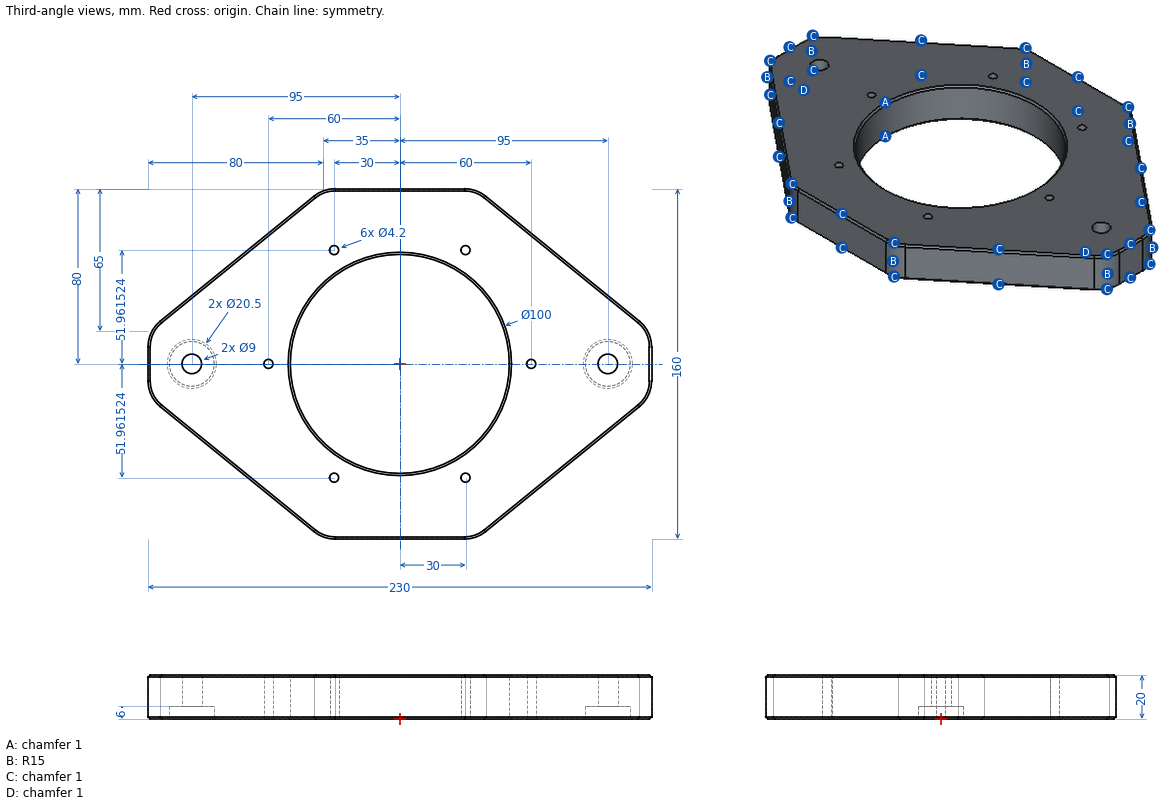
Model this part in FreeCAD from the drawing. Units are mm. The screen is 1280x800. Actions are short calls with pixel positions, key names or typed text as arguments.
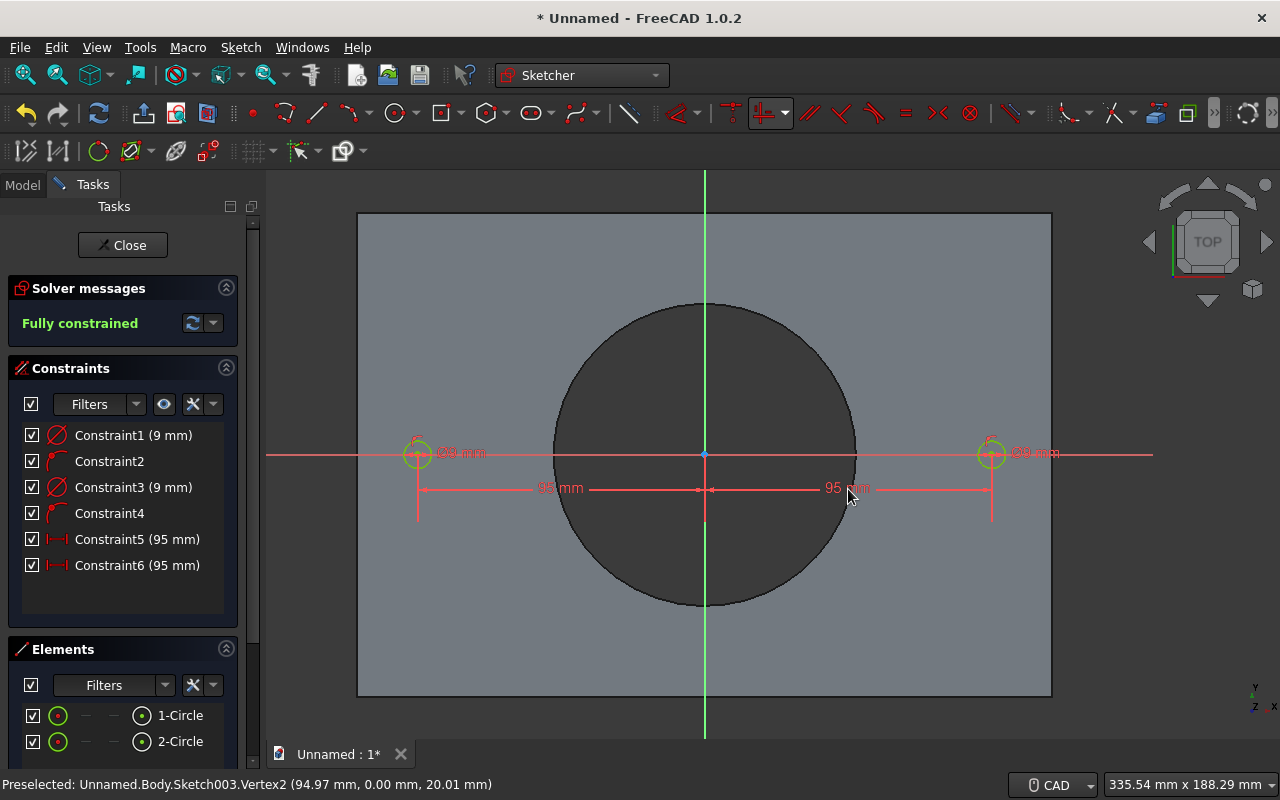
click(123, 245)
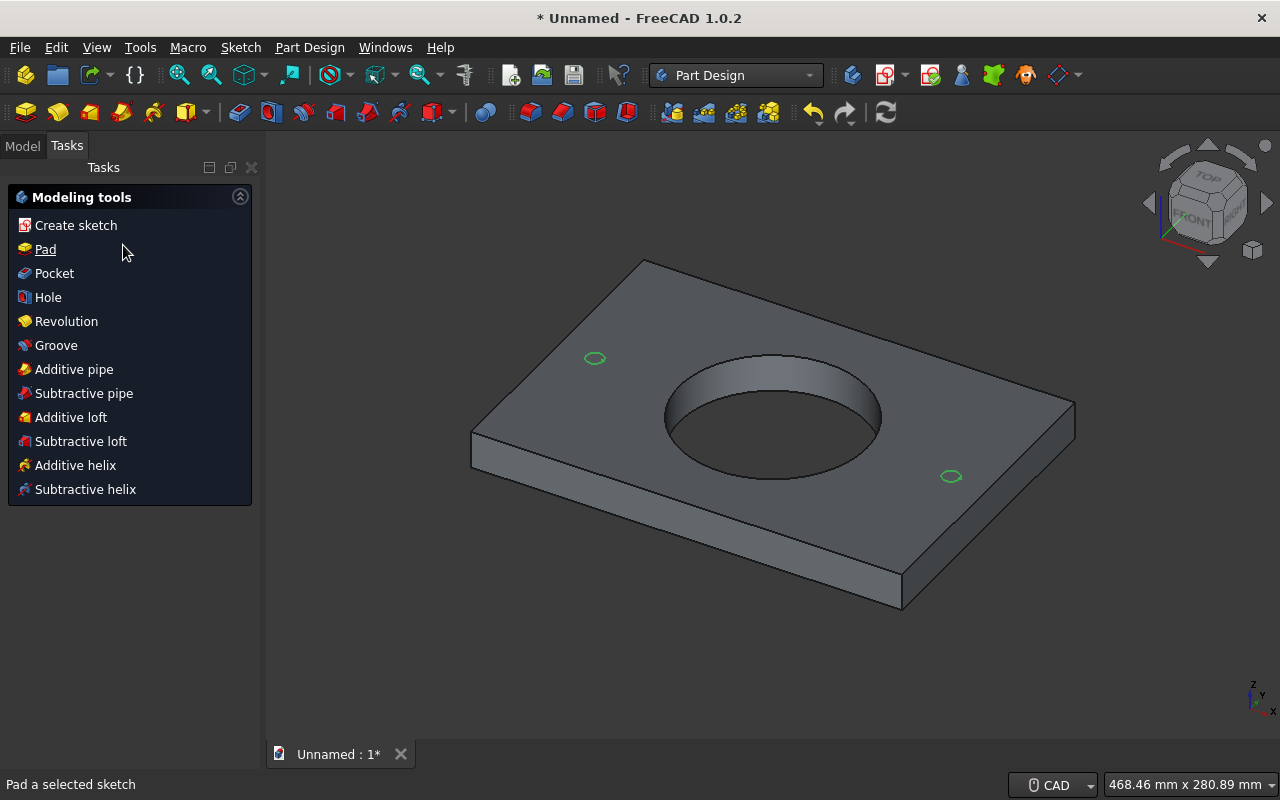
click(240, 112)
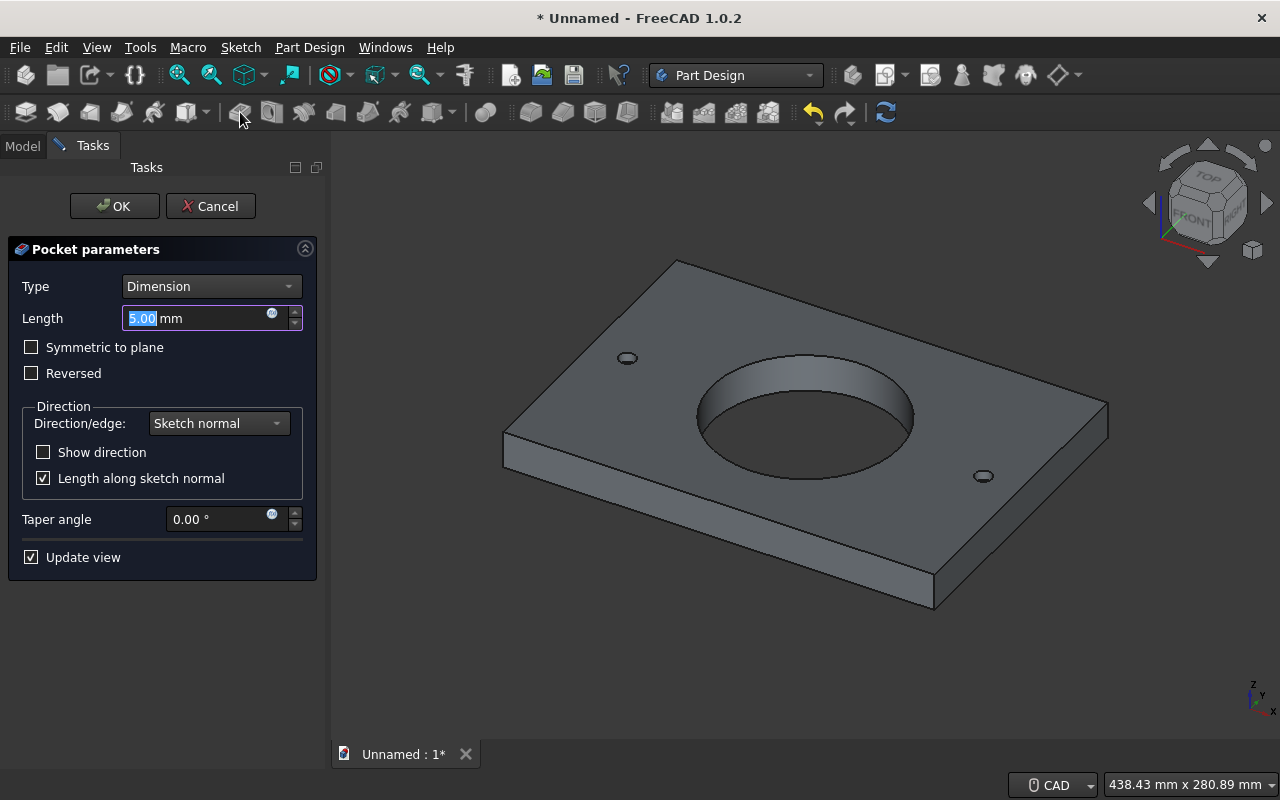
click(212, 286)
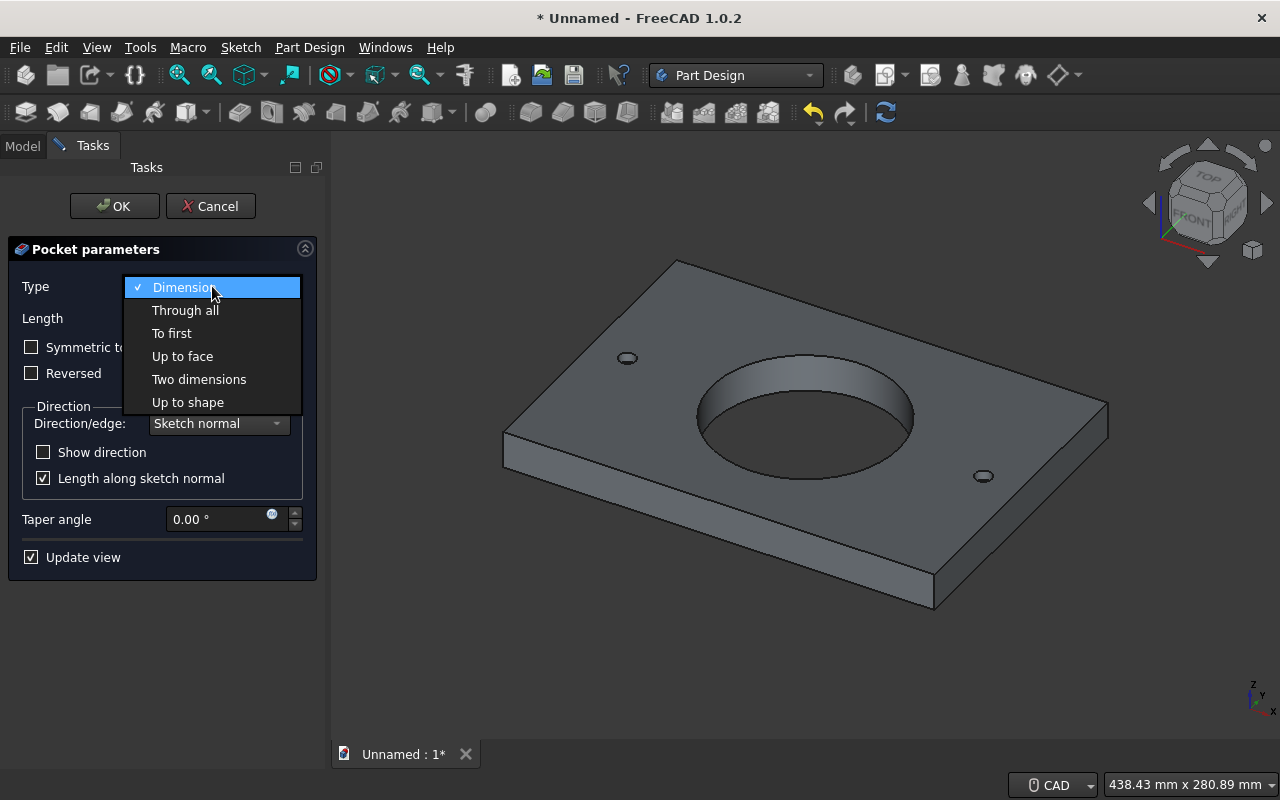
click(212, 310)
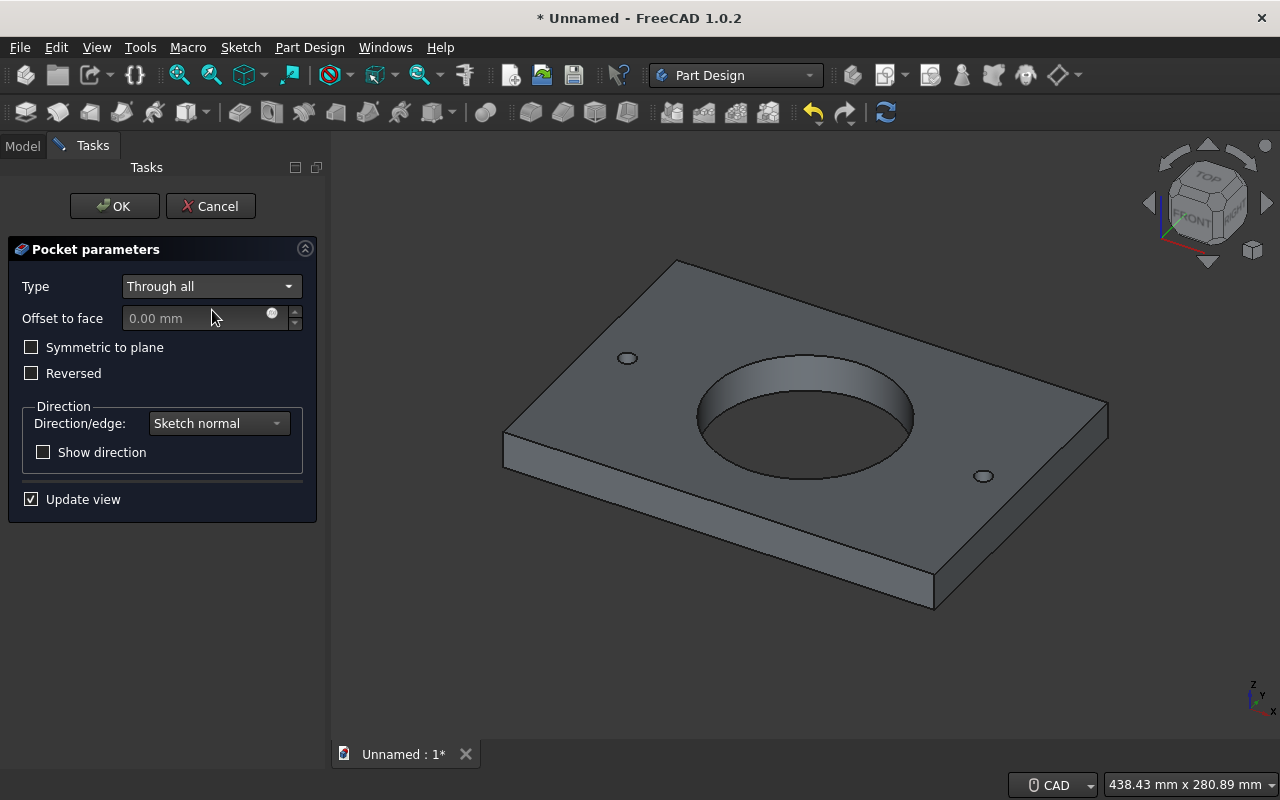
click(115, 206)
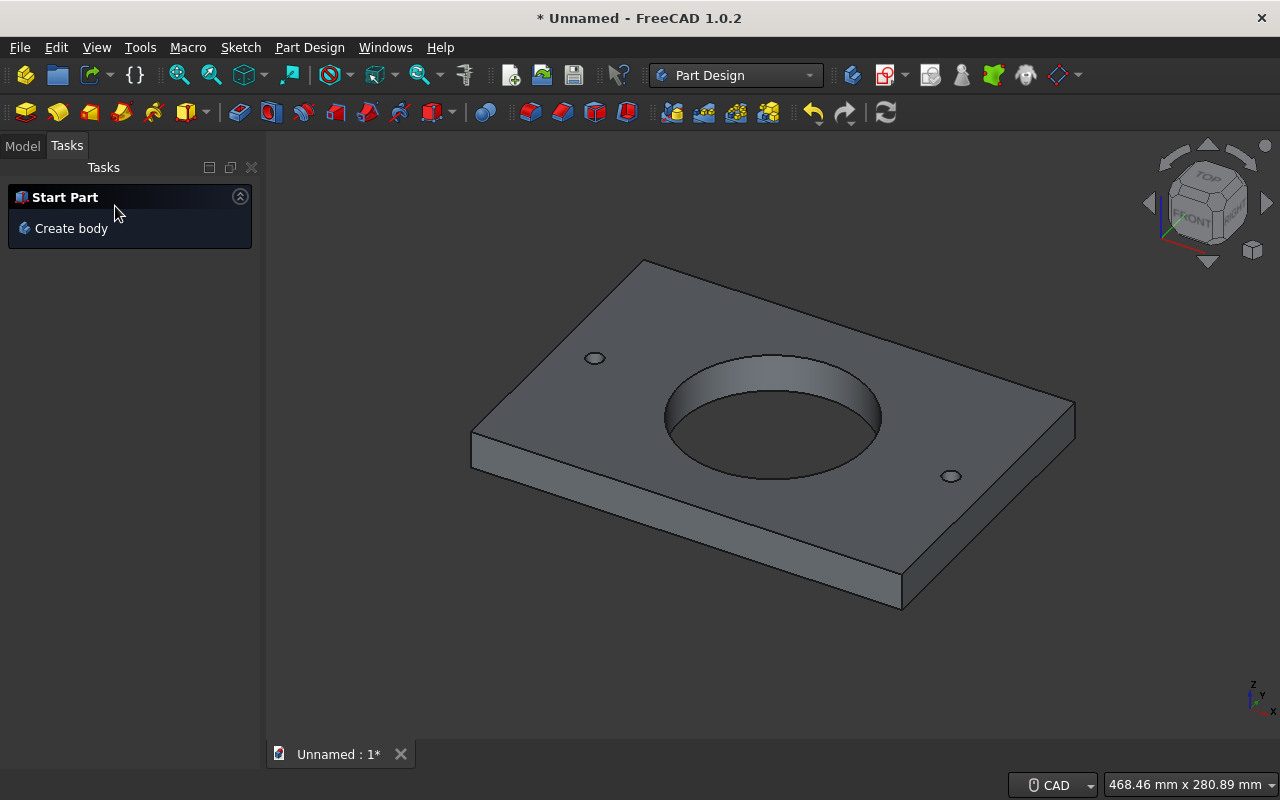
click(679, 385)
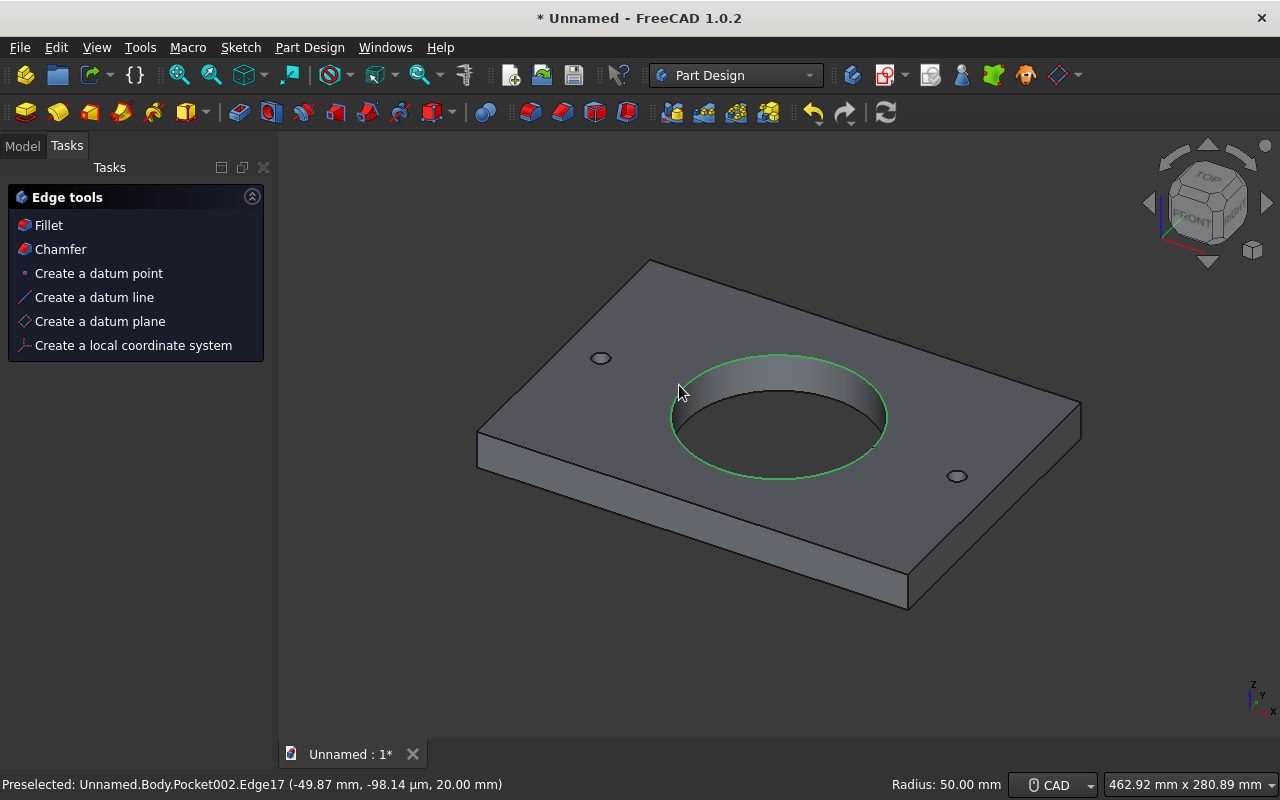
key(0)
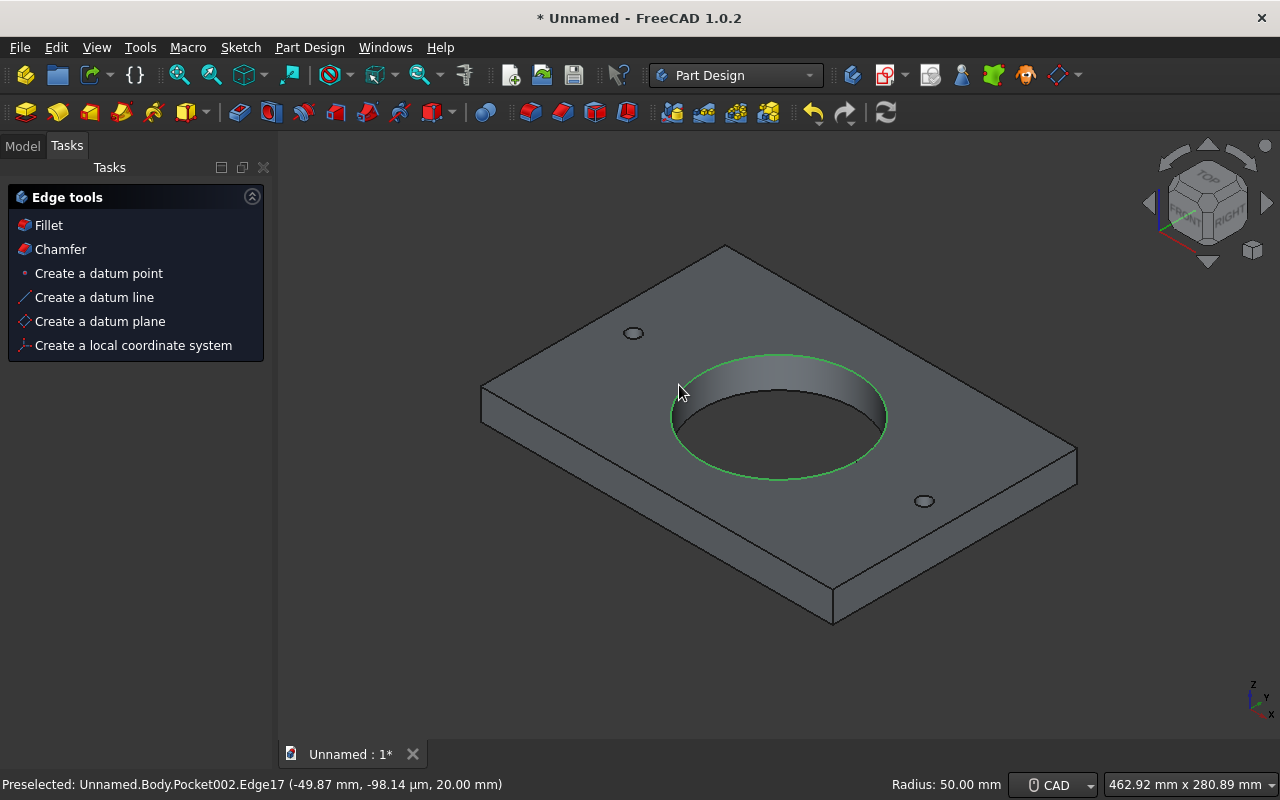
key(2)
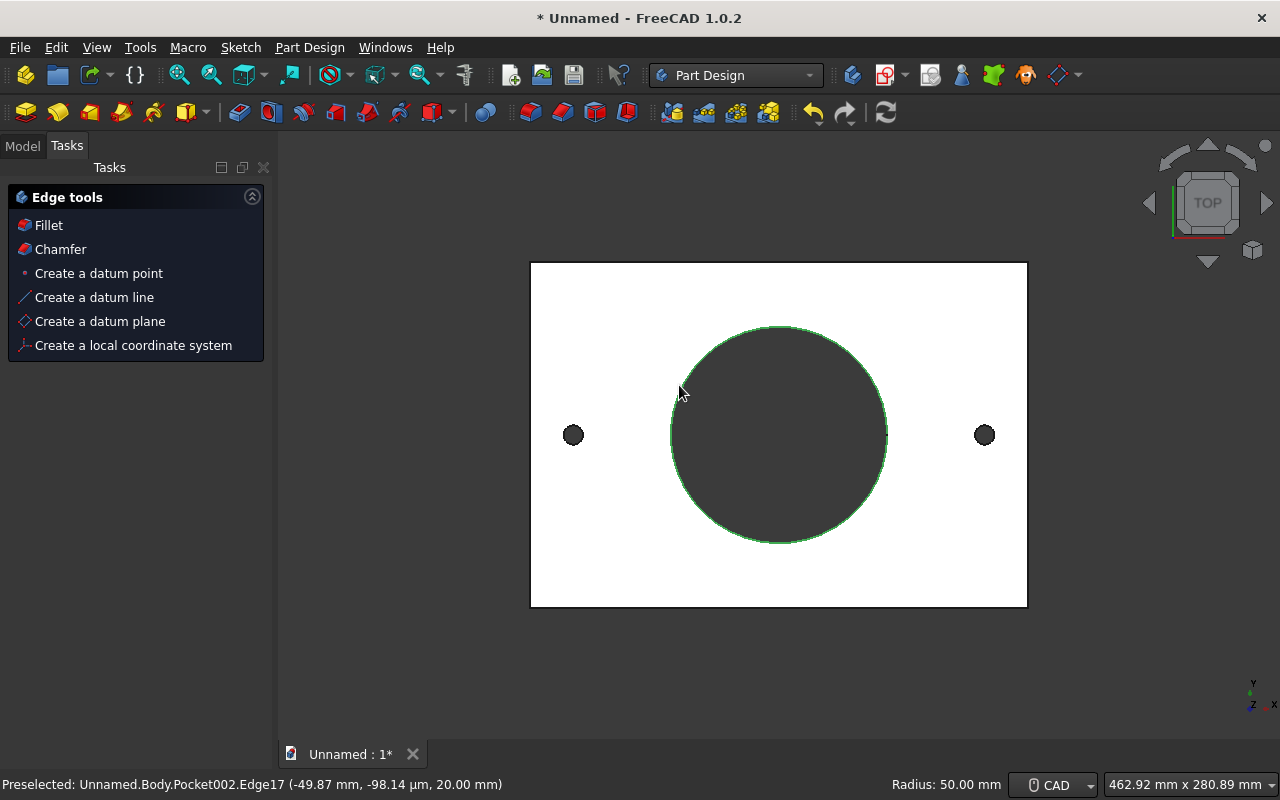
key(1)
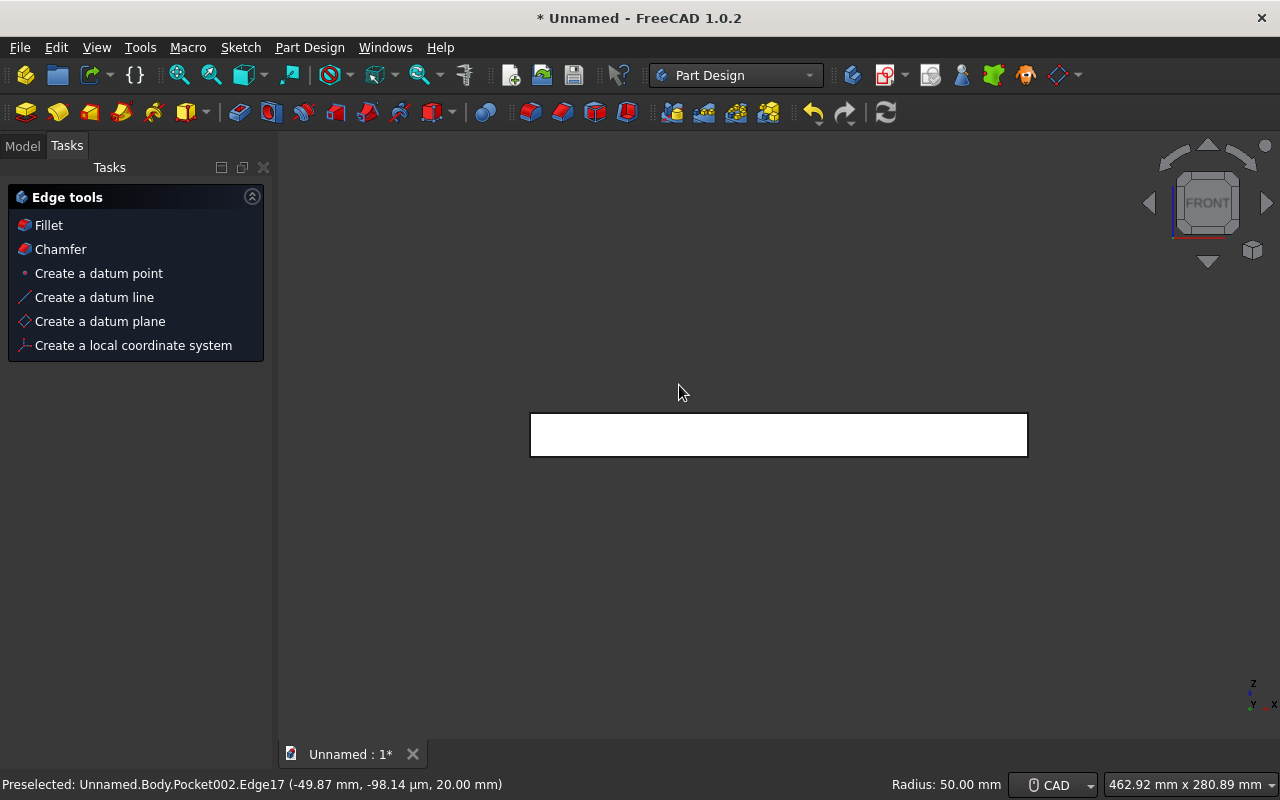
key(3)